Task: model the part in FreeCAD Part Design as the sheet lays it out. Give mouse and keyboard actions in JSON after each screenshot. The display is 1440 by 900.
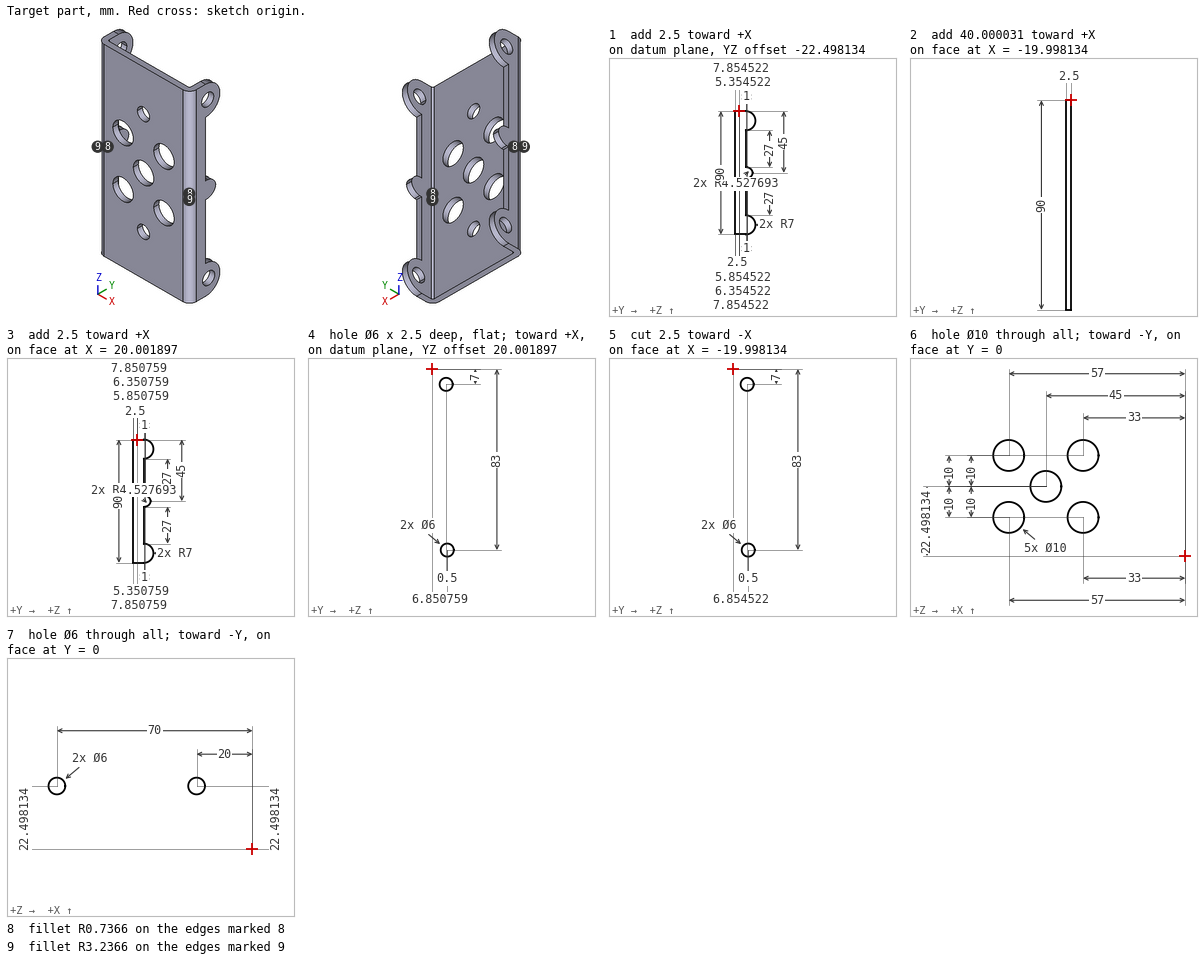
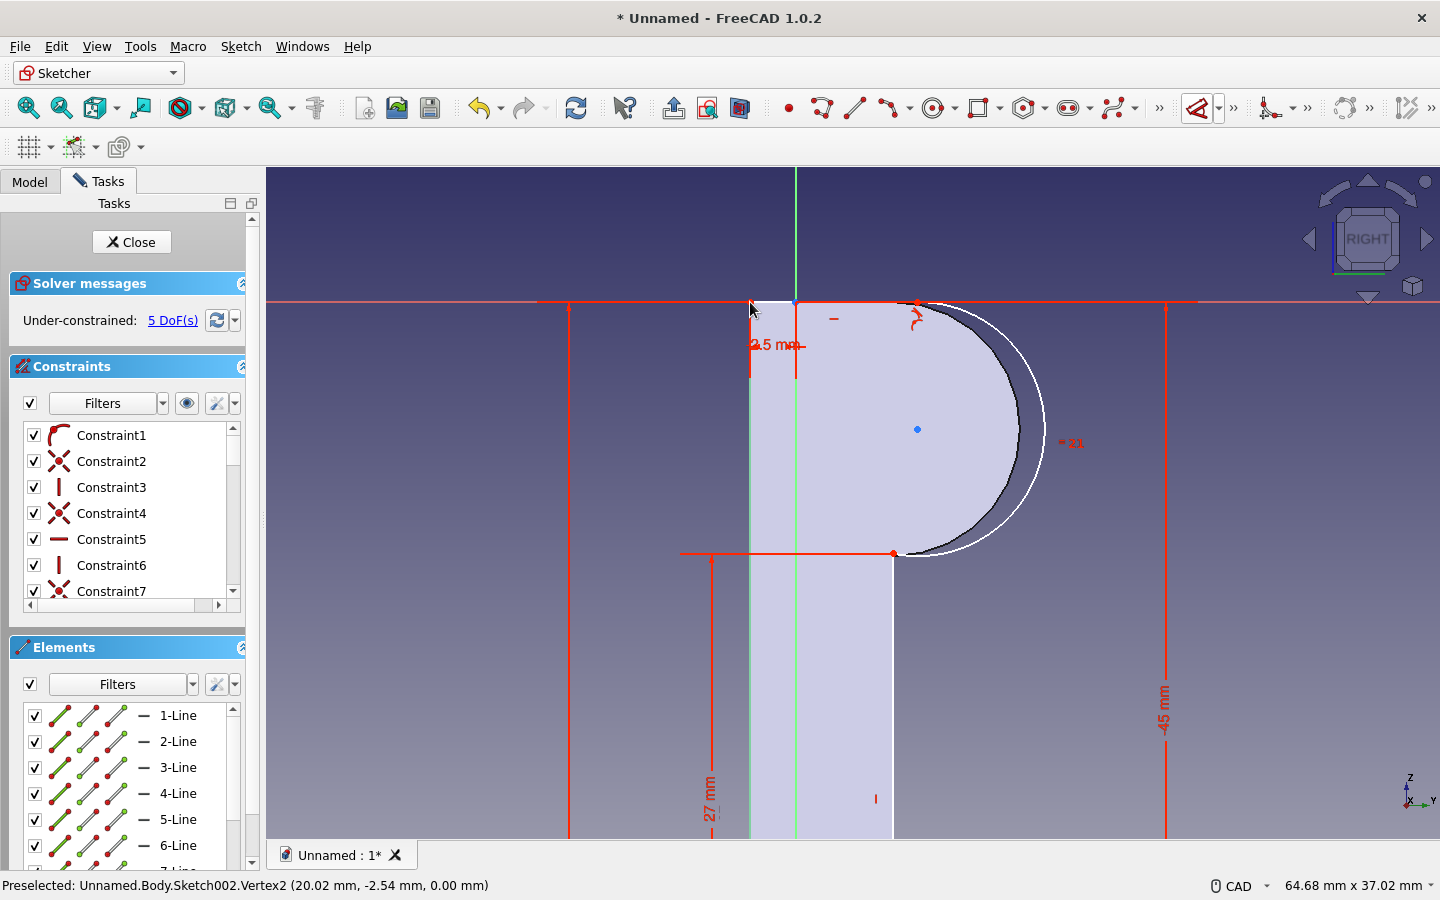
{"action": "scroll", "coordinate": [752, 301], "scroll_direction": "down", "scroll_amount": 7}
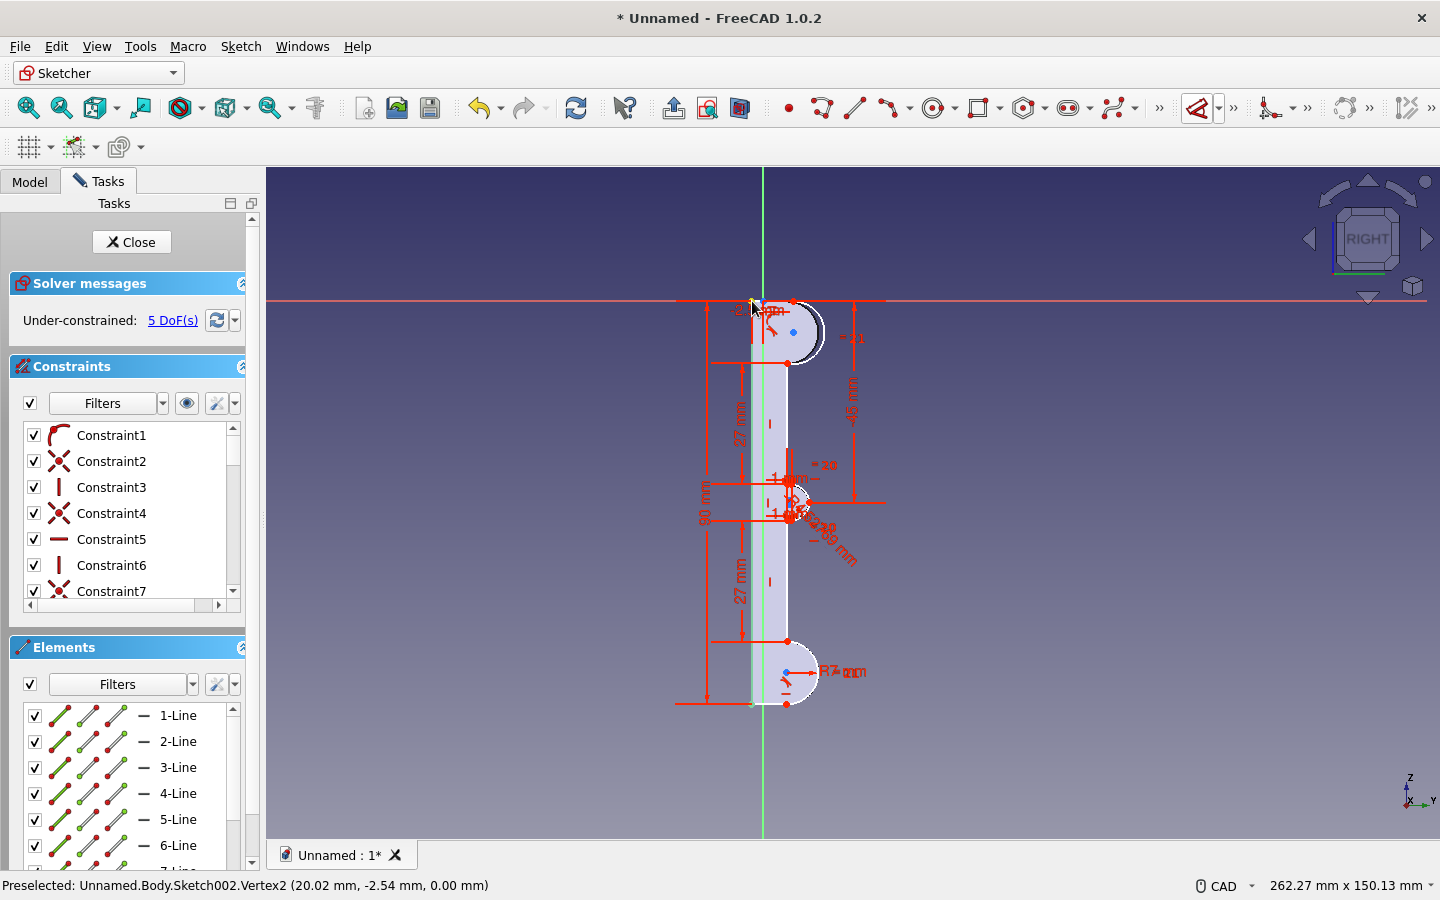
{"action": "left_click", "coordinate": [781, 301]}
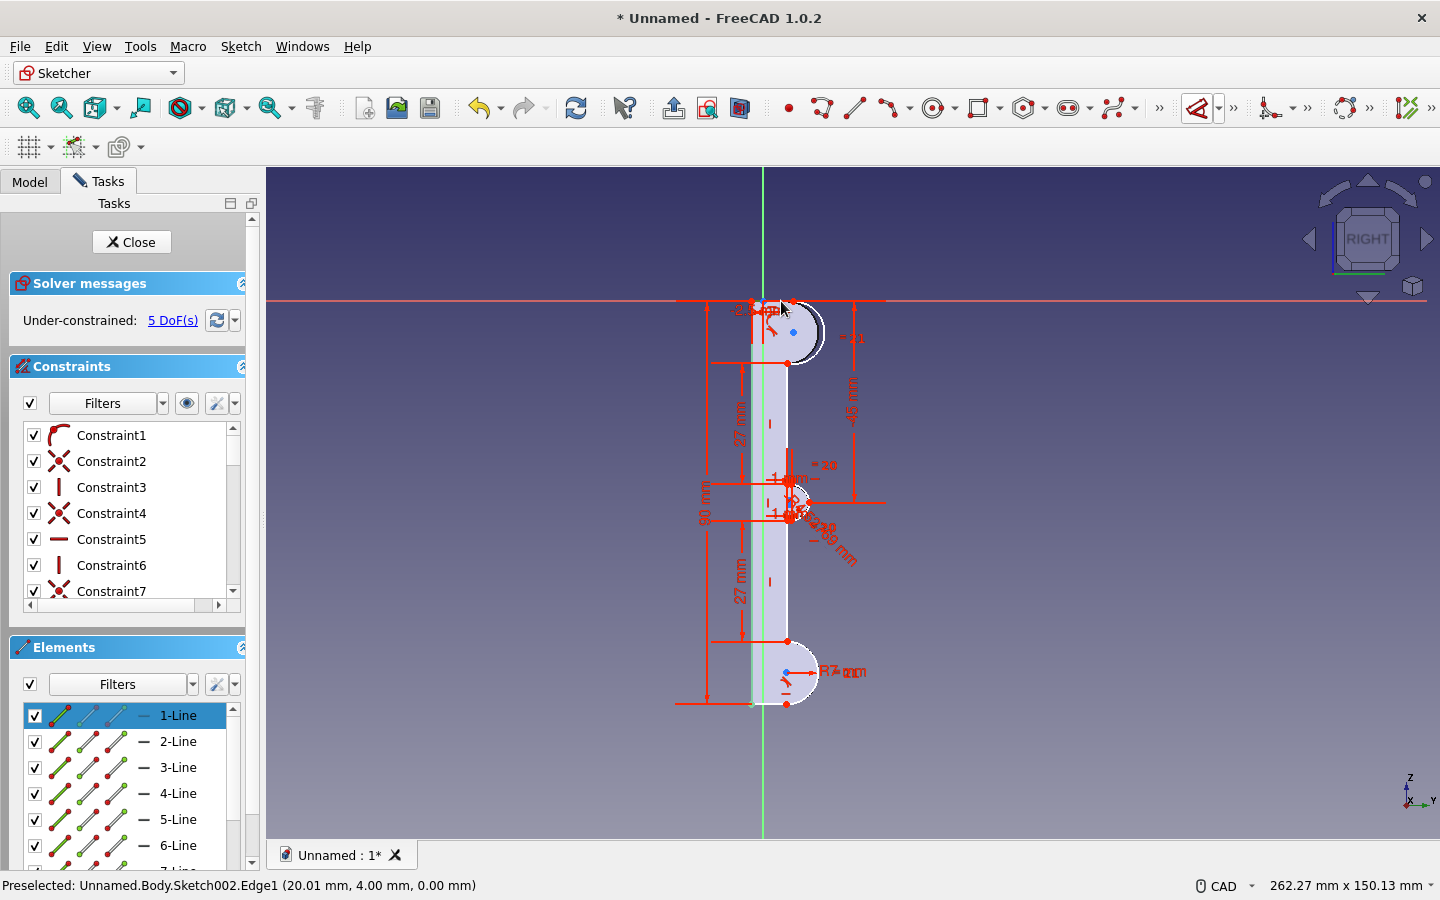
{"action": "left_click", "coordinate": [1218, 108]}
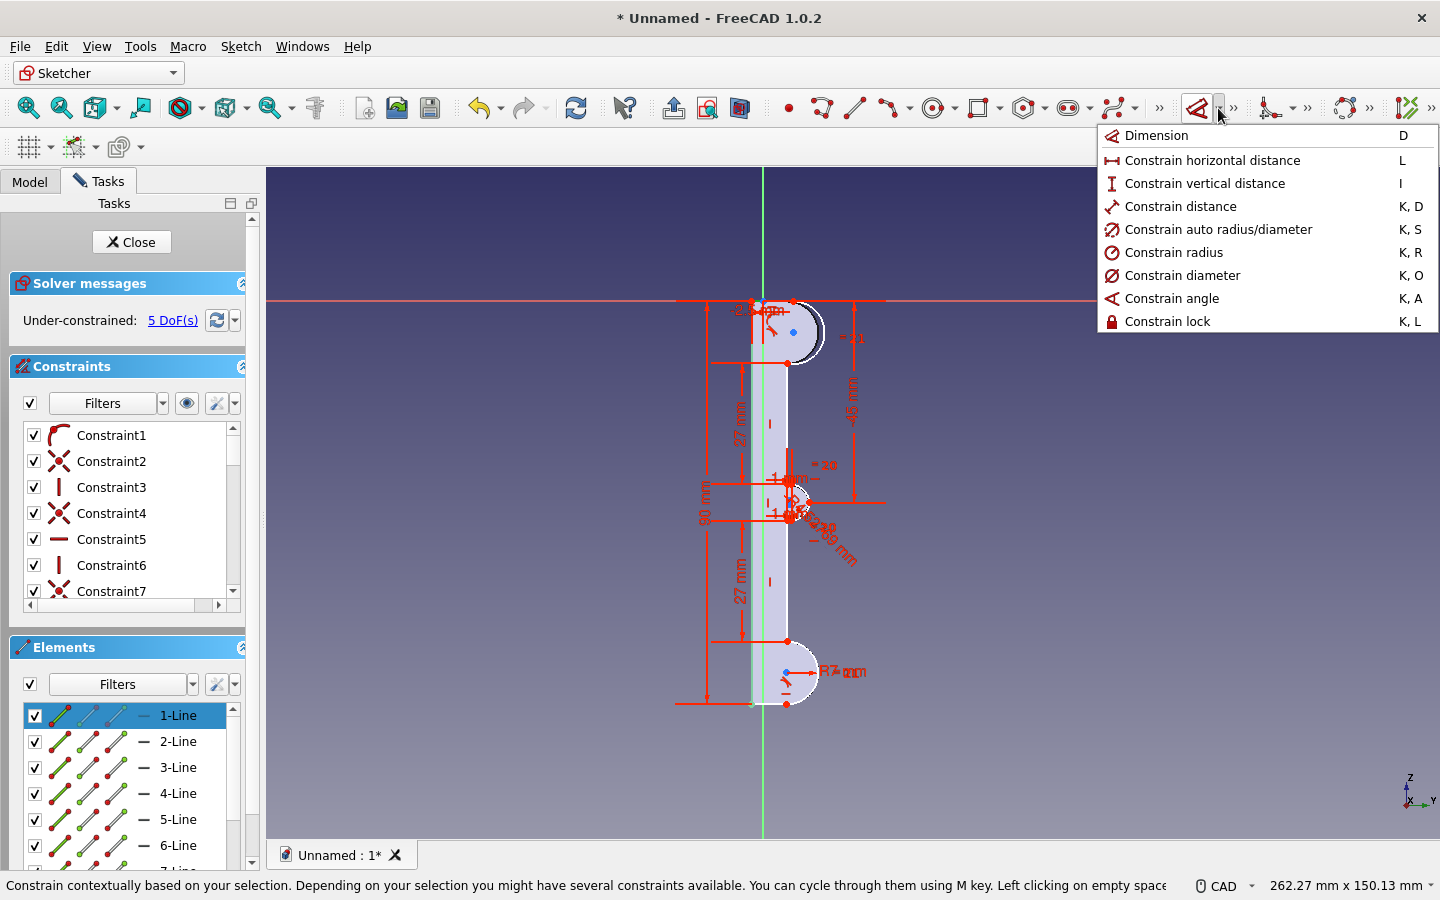
{"action": "left_click", "coordinate": [1268, 160]}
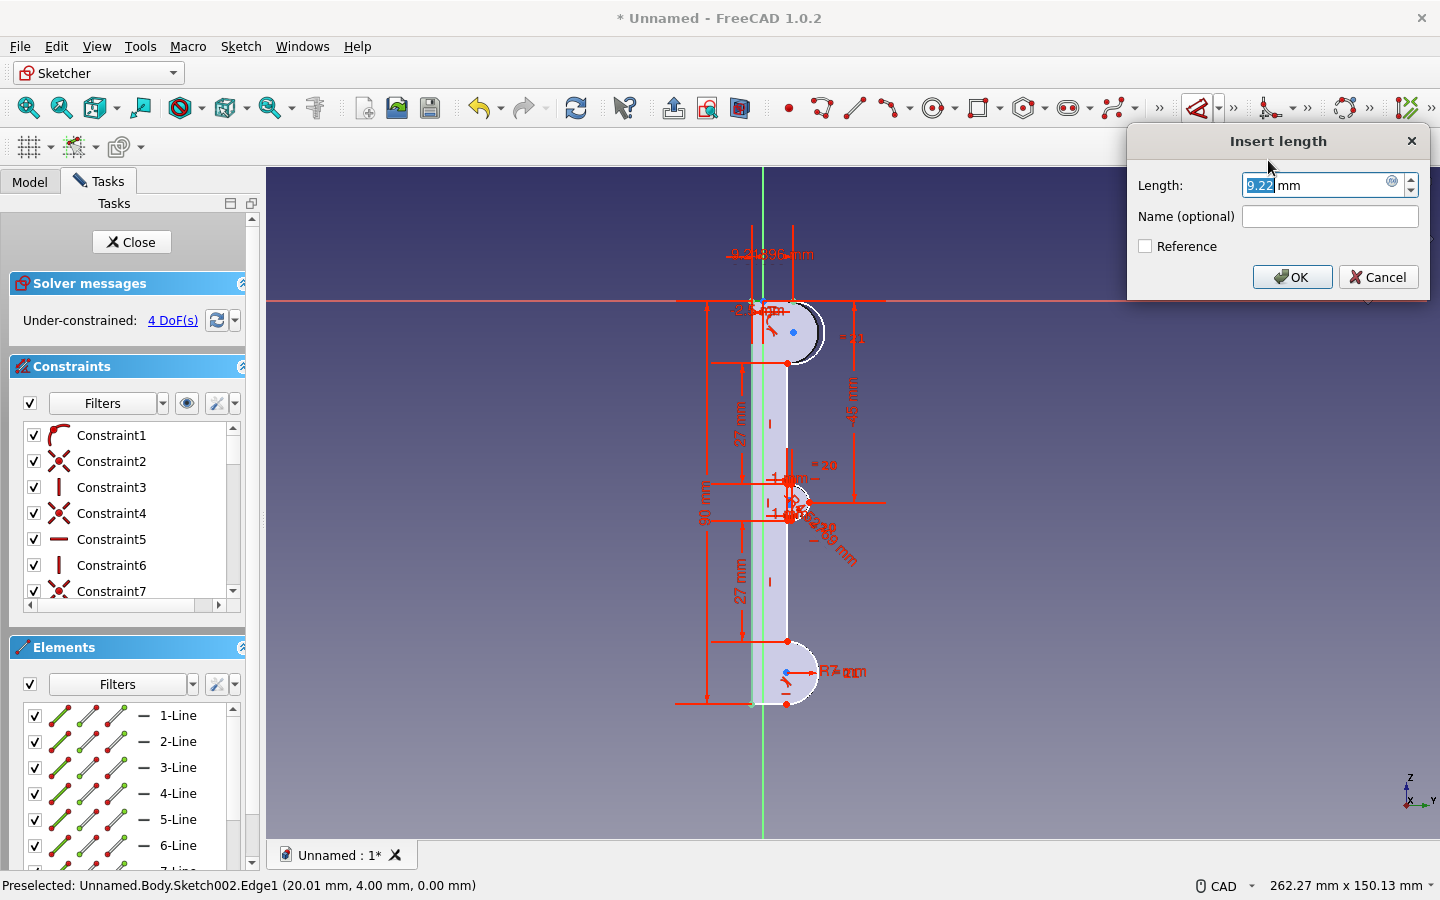
{"action": "type", "text": "7.850759"}
{"action": "key", "text": "Return"}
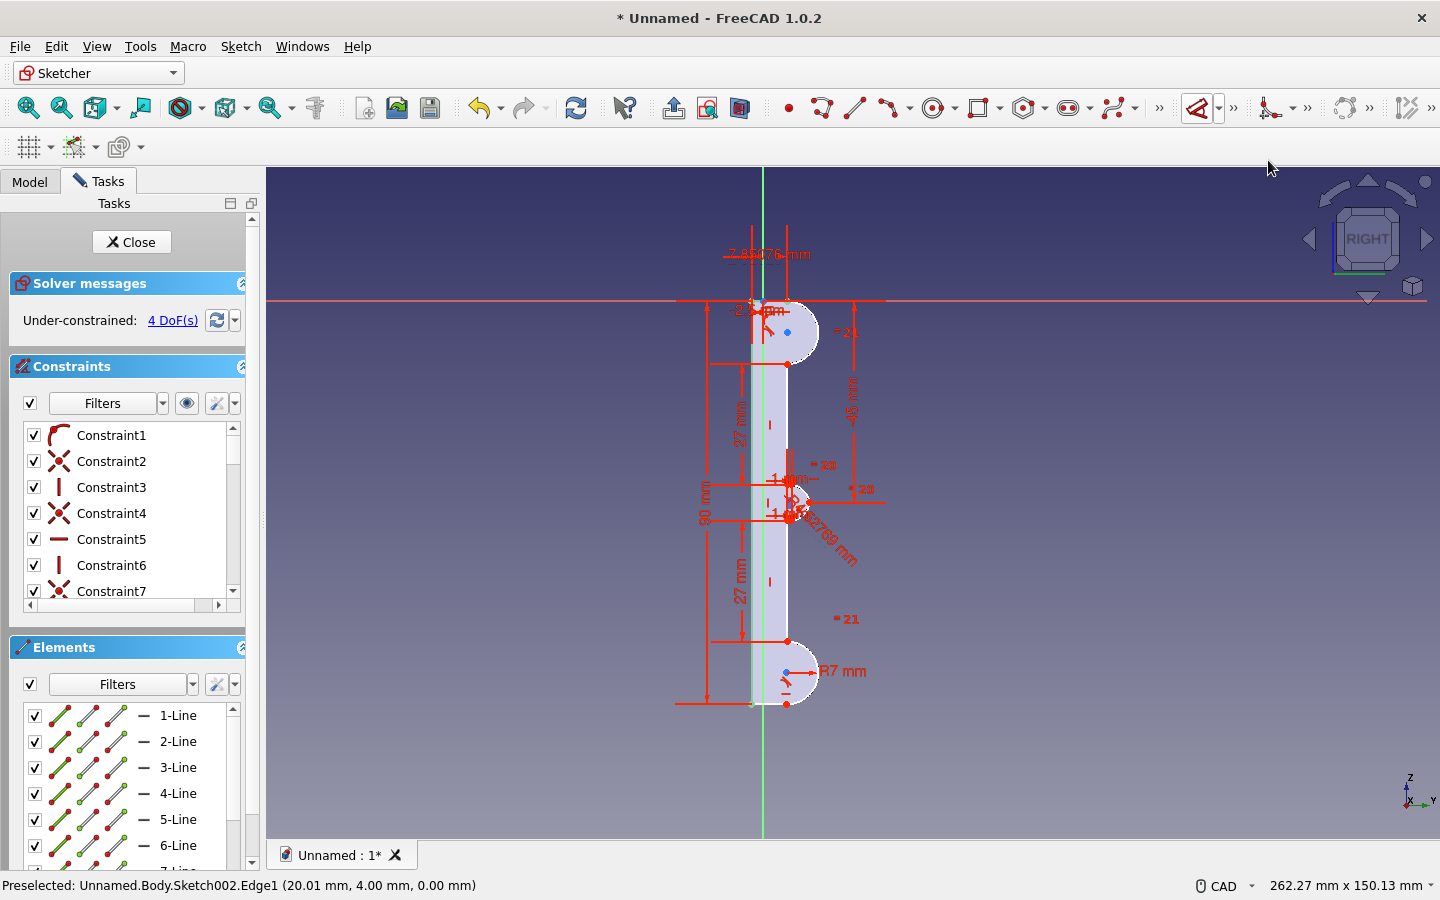
{"action": "scroll", "coordinate": [762, 704], "scroll_direction": "up", "scroll_amount": 2}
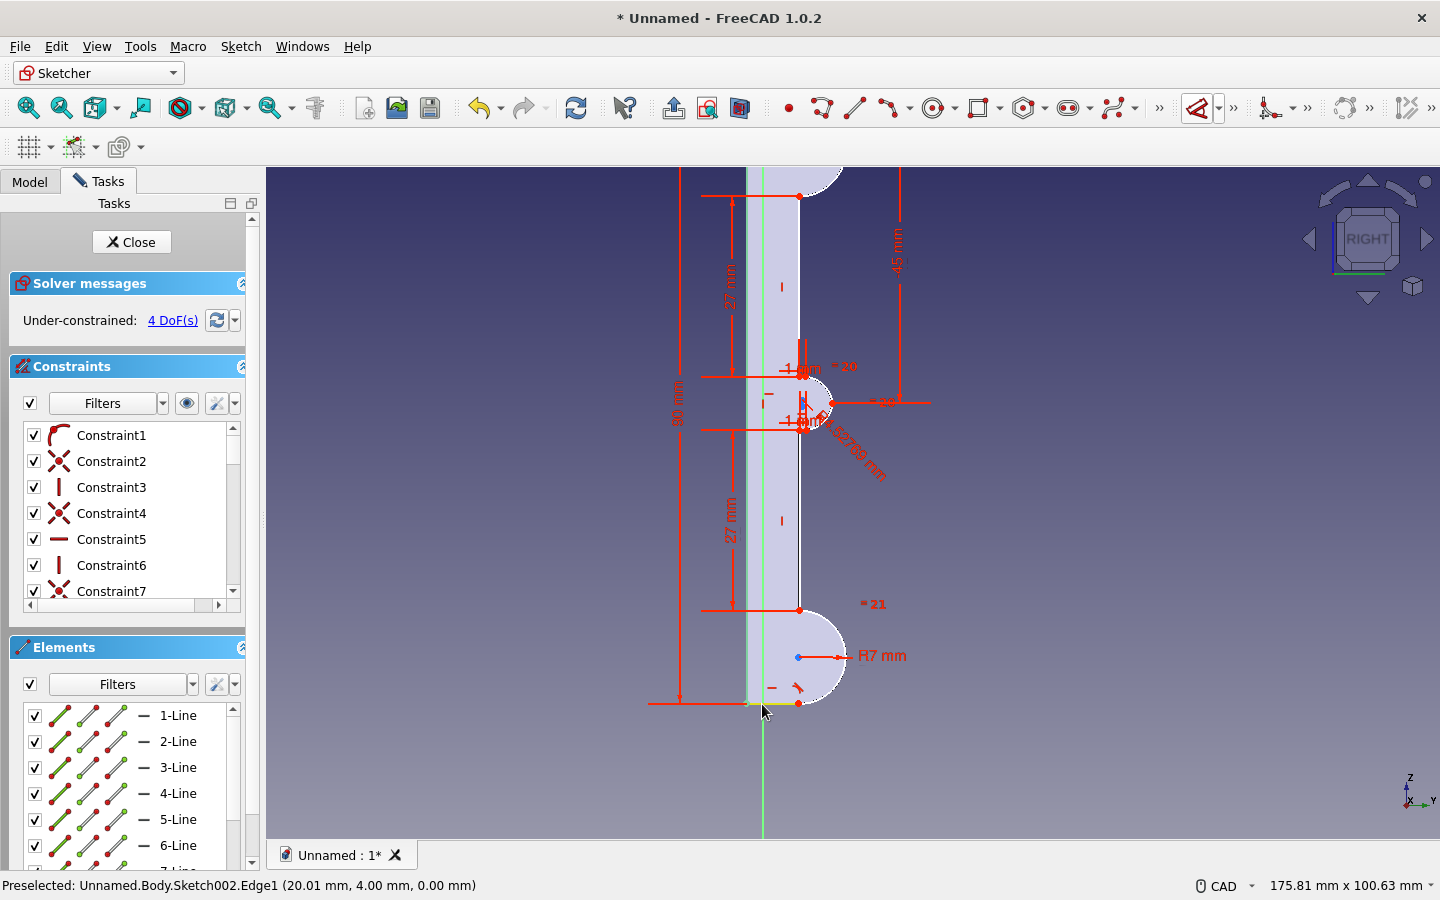
{"action": "left_click", "coordinate": [762, 704]}